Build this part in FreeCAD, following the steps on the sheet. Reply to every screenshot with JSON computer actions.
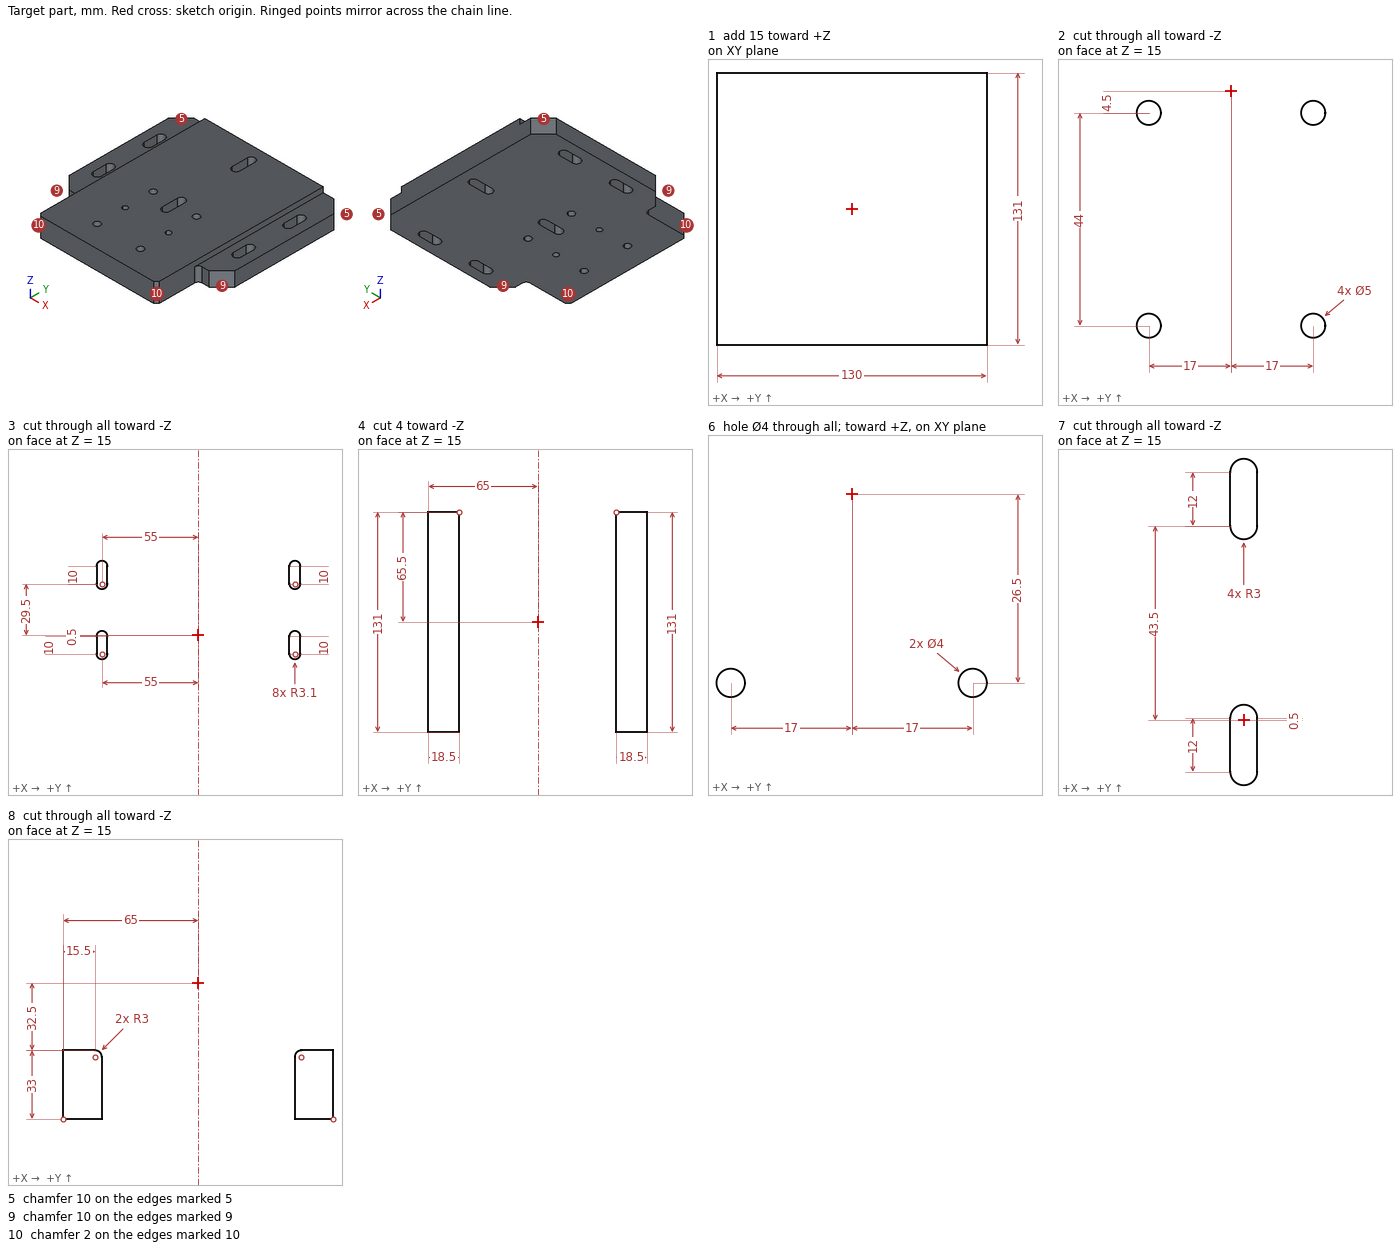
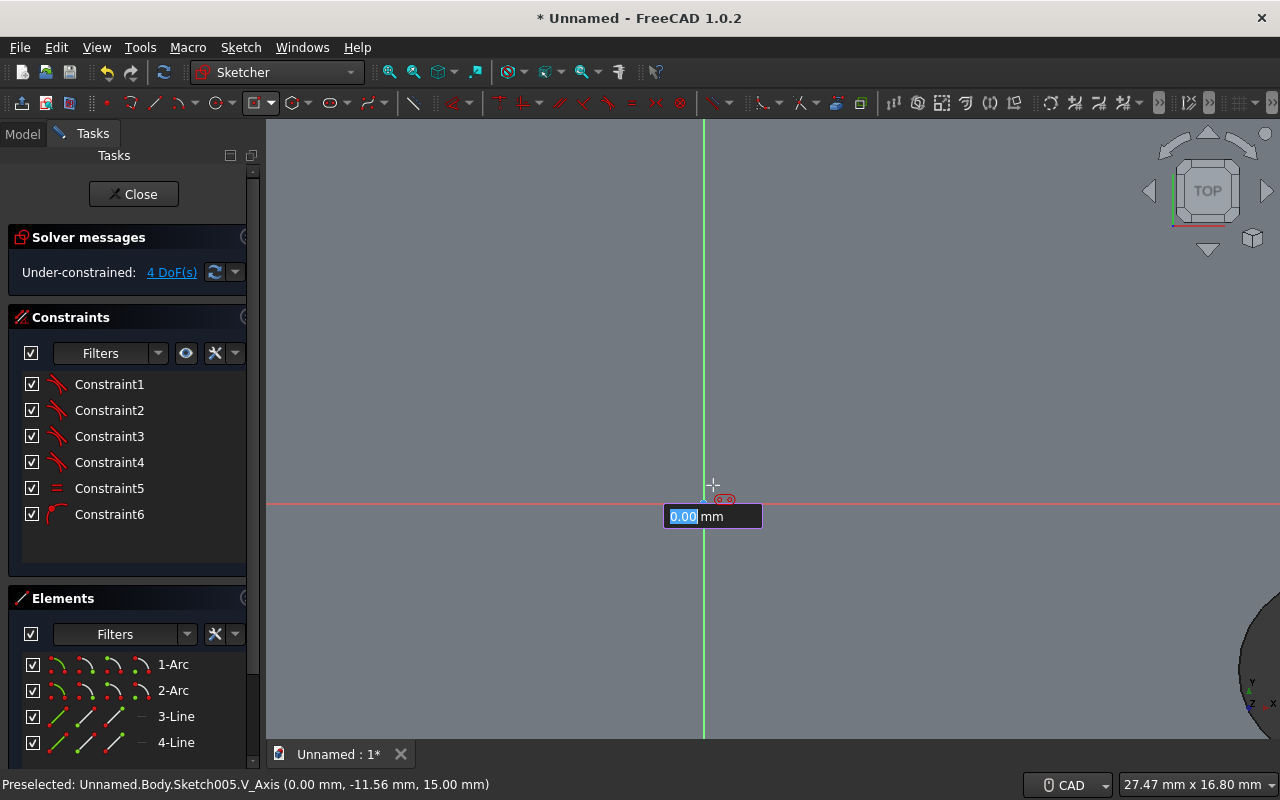
{"action": "scroll", "coordinate": [705, 544], "scroll_direction": "down", "scroll_amount": 10}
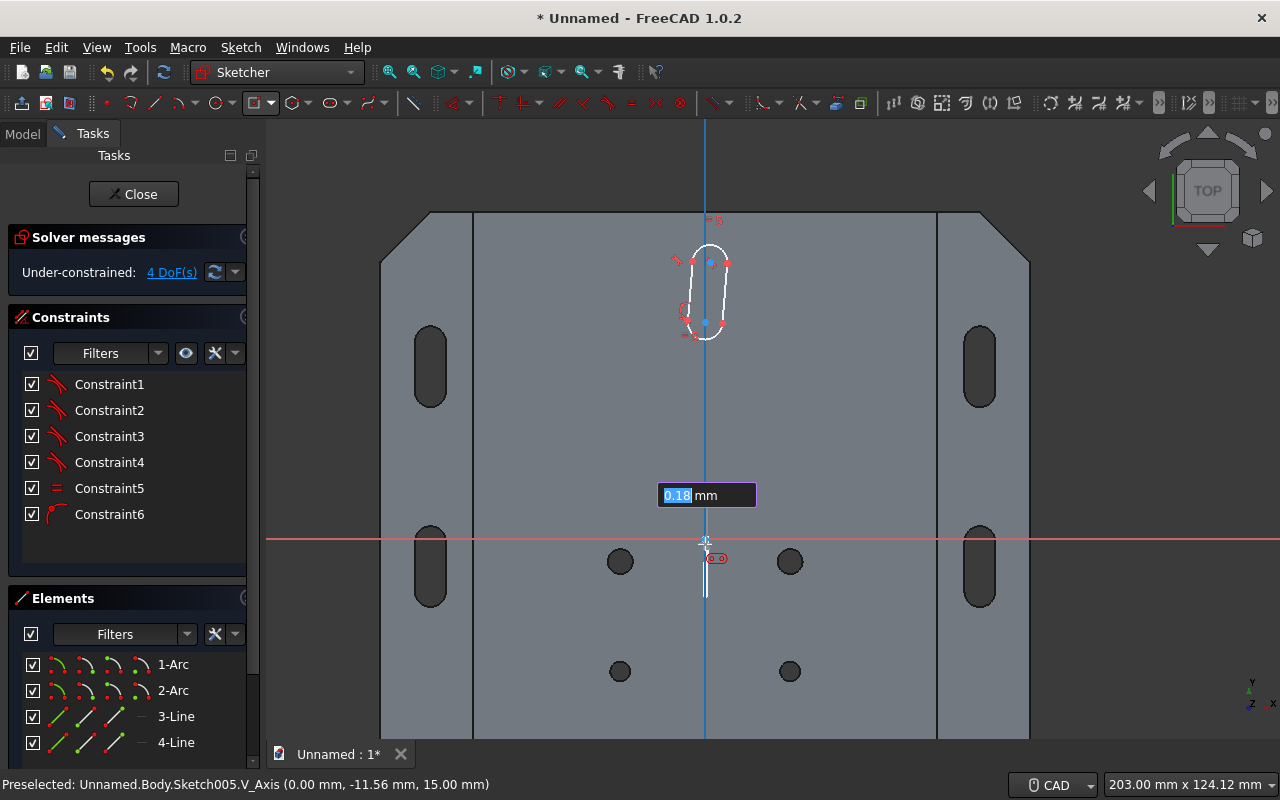
{"action": "left_click", "coordinate": [720, 567]}
{"action": "key", "text": "Escape"}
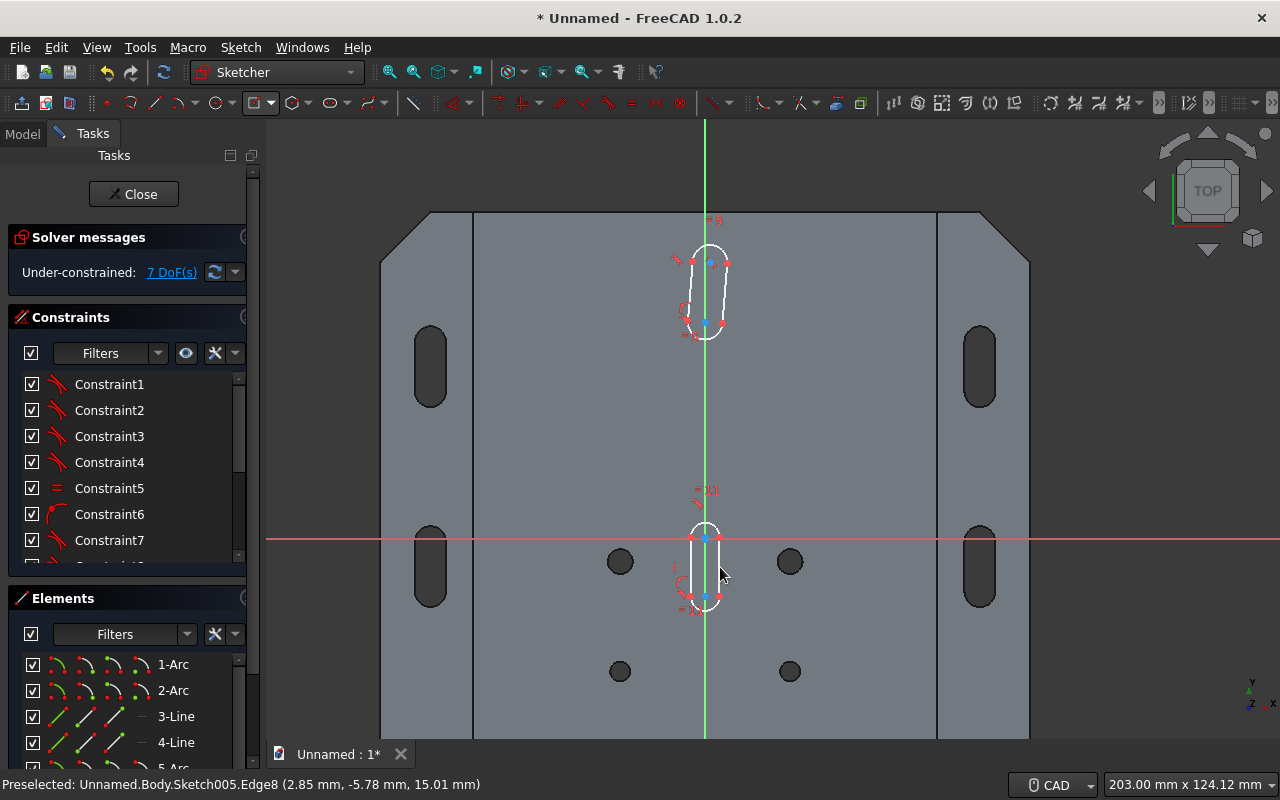
{"action": "left_click", "coordinate": [691, 279]}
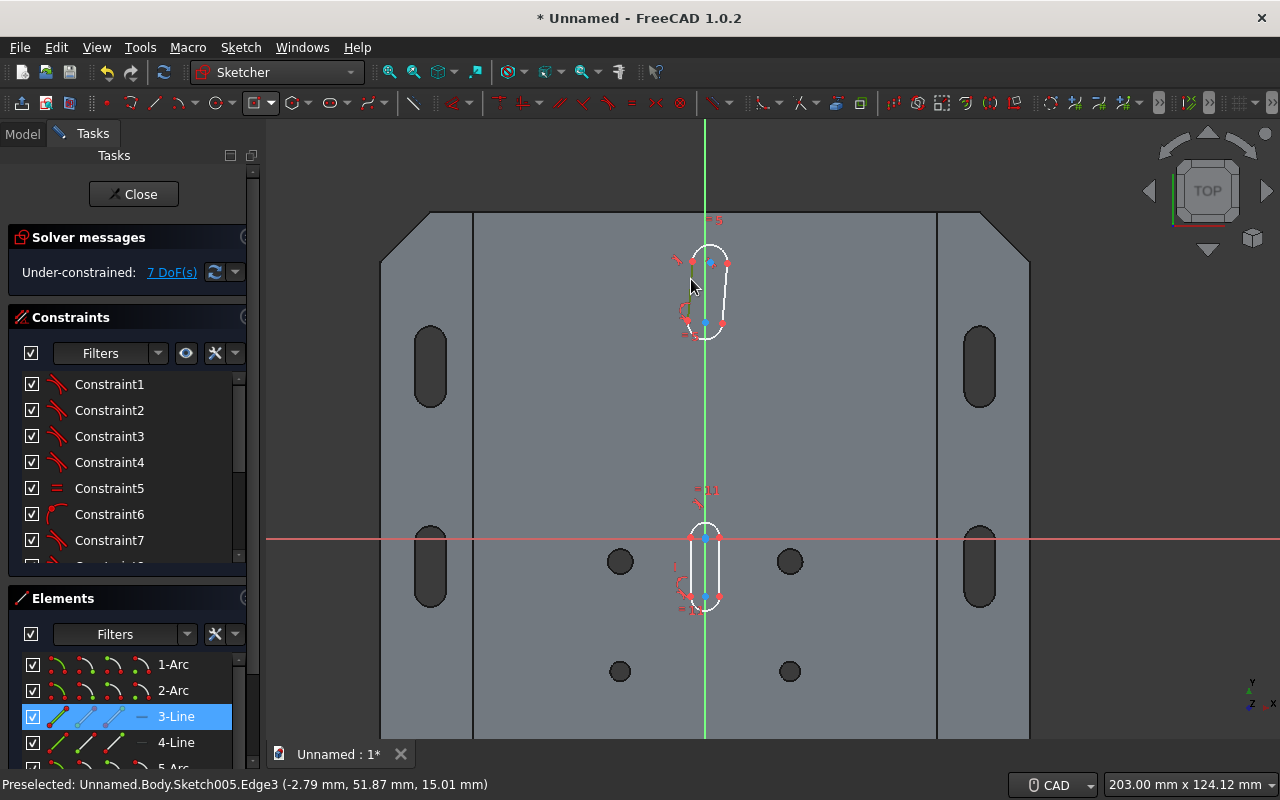
{"action": "key", "text": "v"}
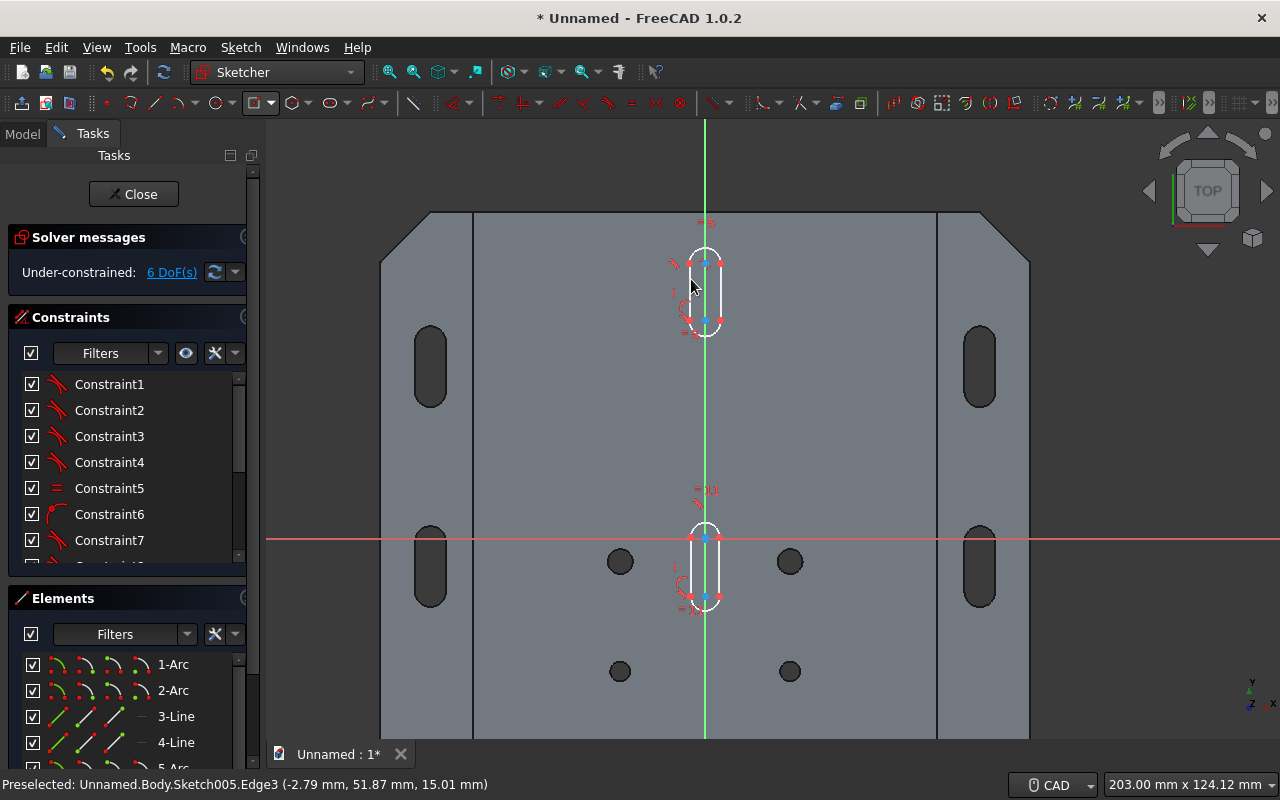
{"action": "scroll", "coordinate": [696, 334], "scroll_direction": "up", "scroll_amount": 3}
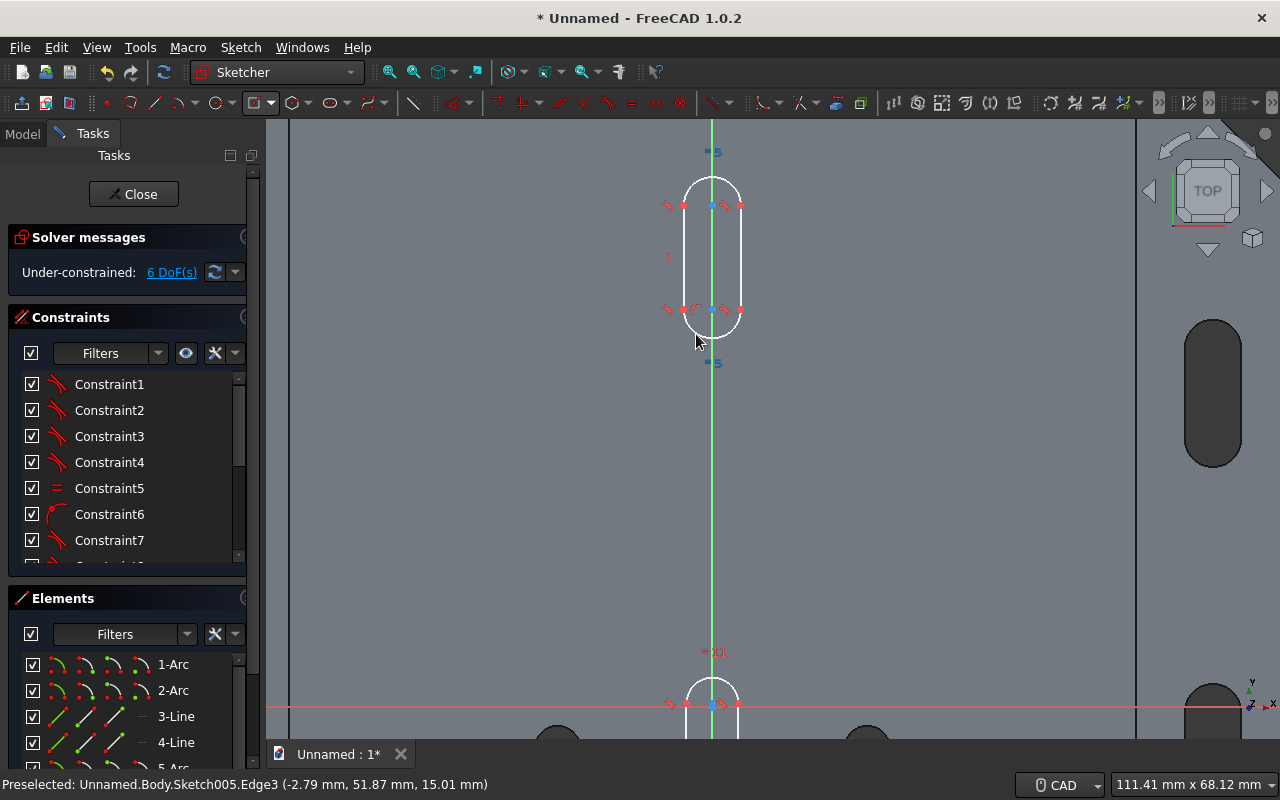
{"action": "left_click", "coordinate": [696, 333]}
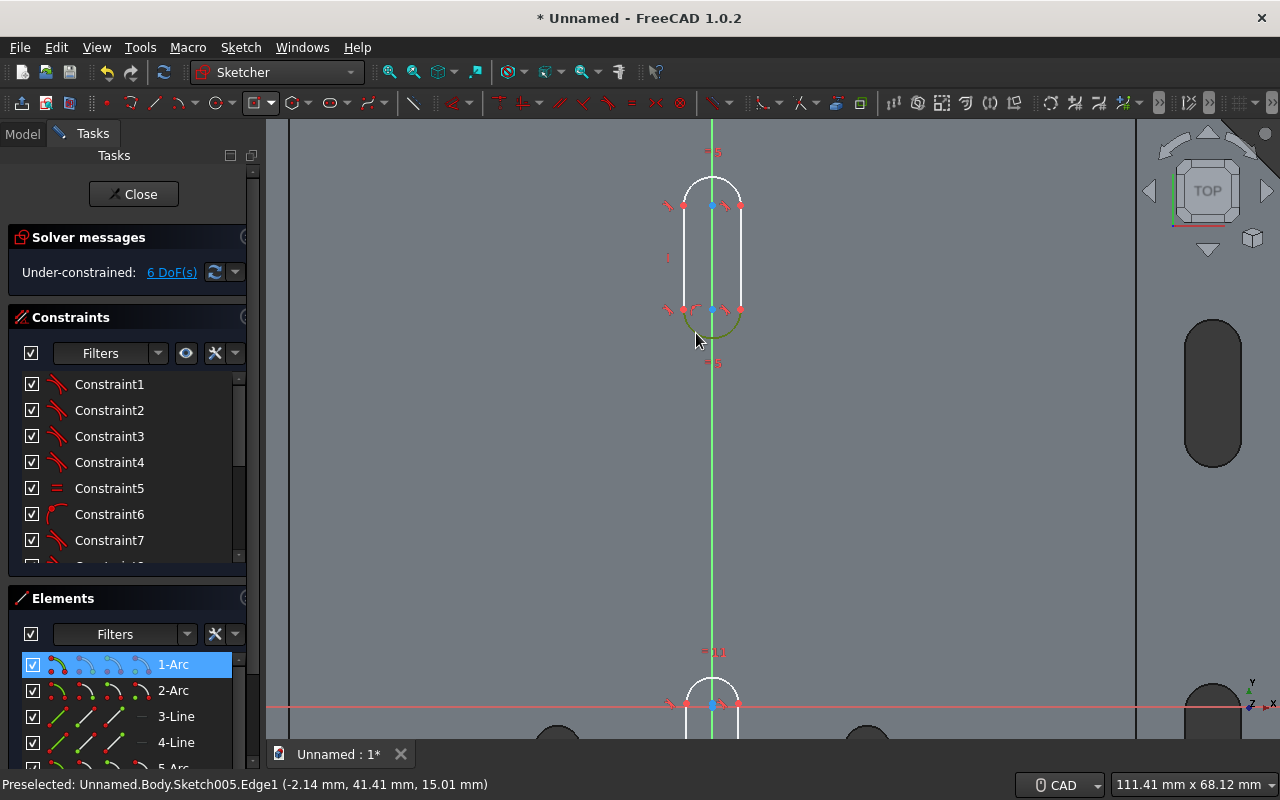
{"action": "scroll", "coordinate": [695, 334], "scroll_direction": "down", "scroll_amount": 3}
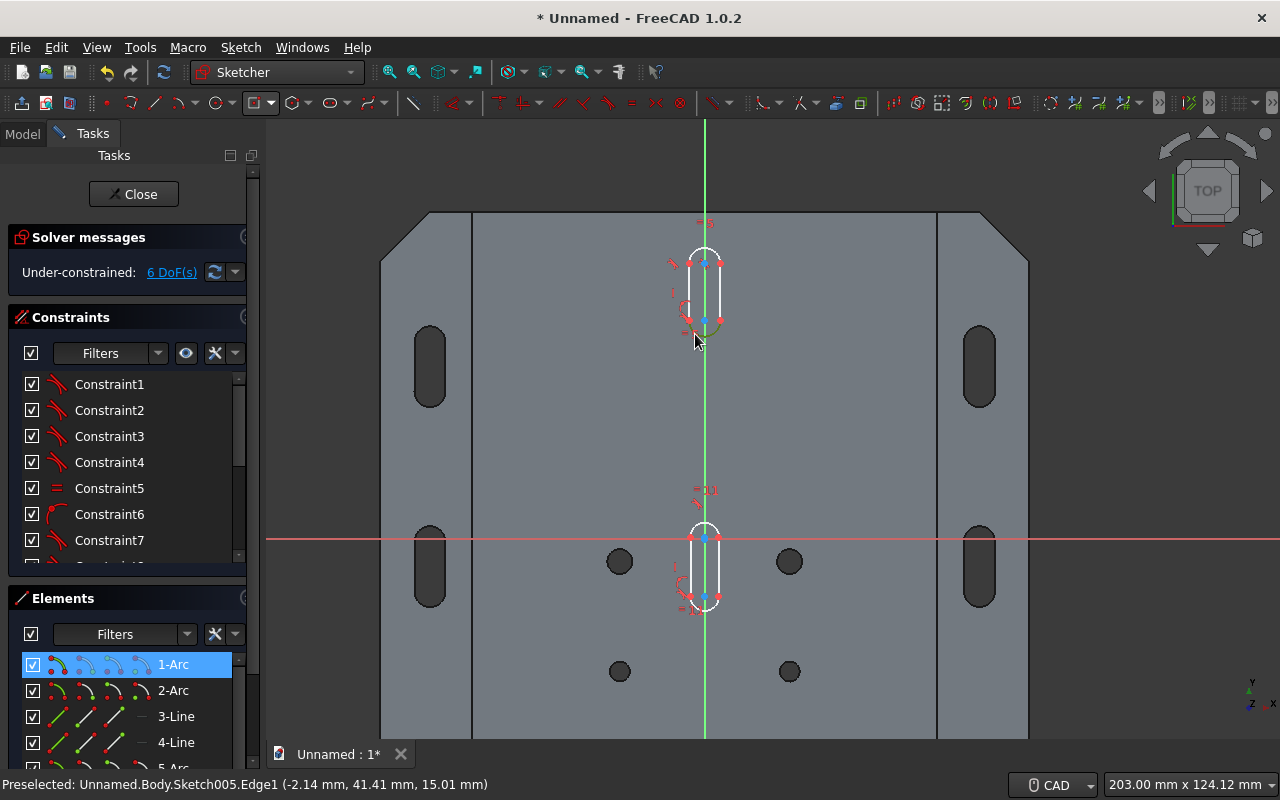
{"action": "scroll", "coordinate": [696, 608], "scroll_direction": "up", "scroll_amount": 3}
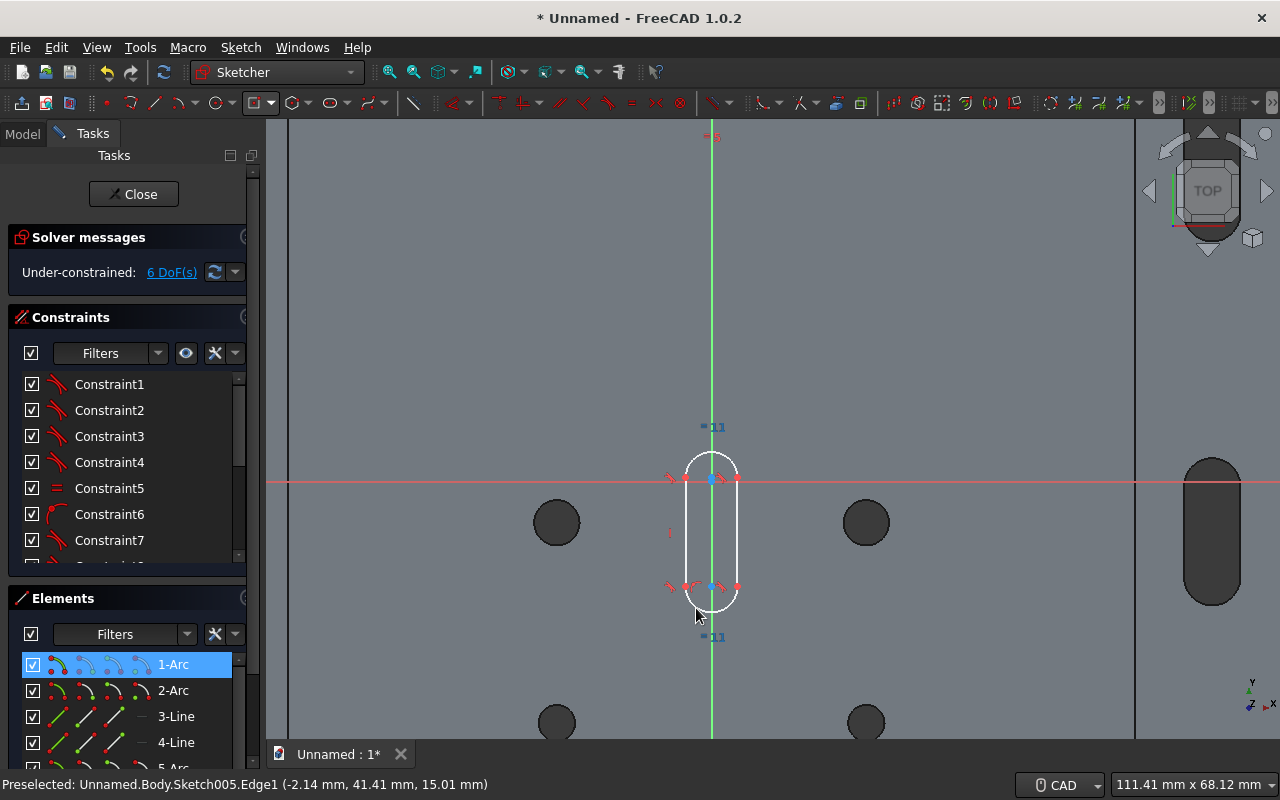
{"action": "left_click", "coordinate": [696, 607]}